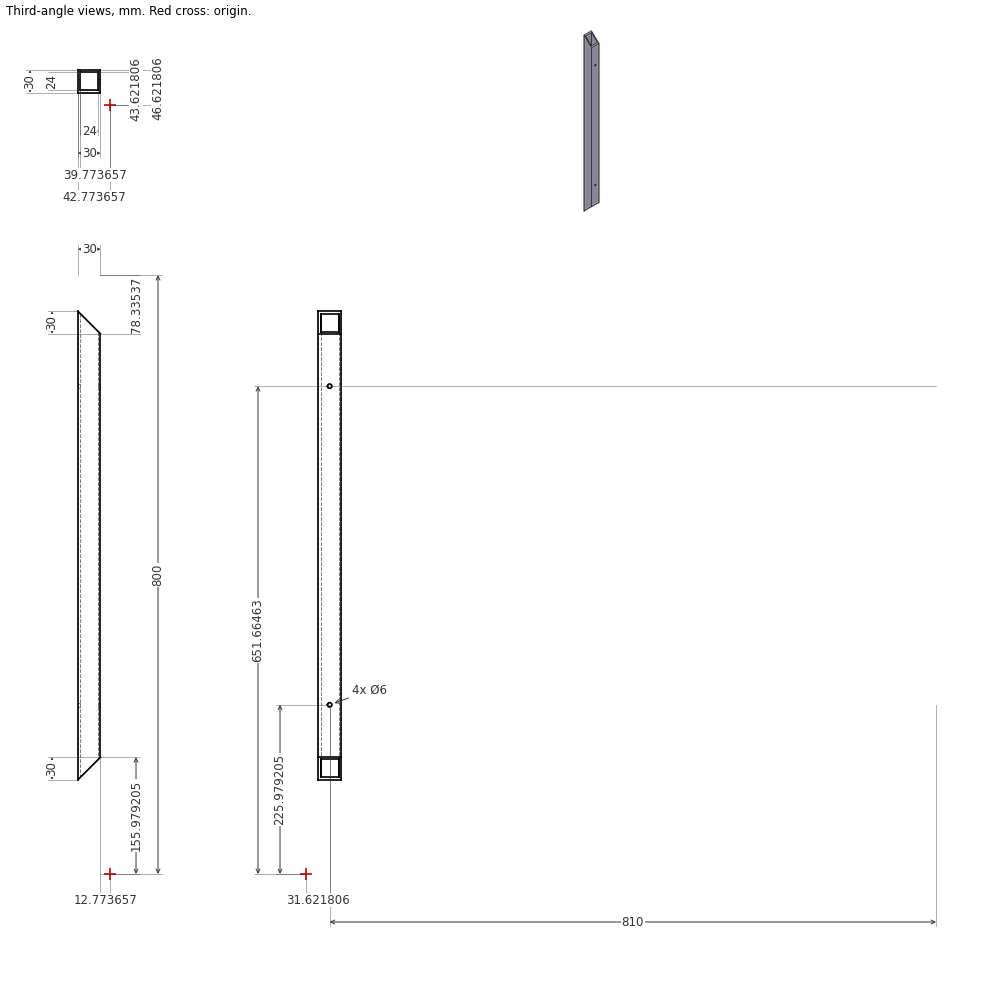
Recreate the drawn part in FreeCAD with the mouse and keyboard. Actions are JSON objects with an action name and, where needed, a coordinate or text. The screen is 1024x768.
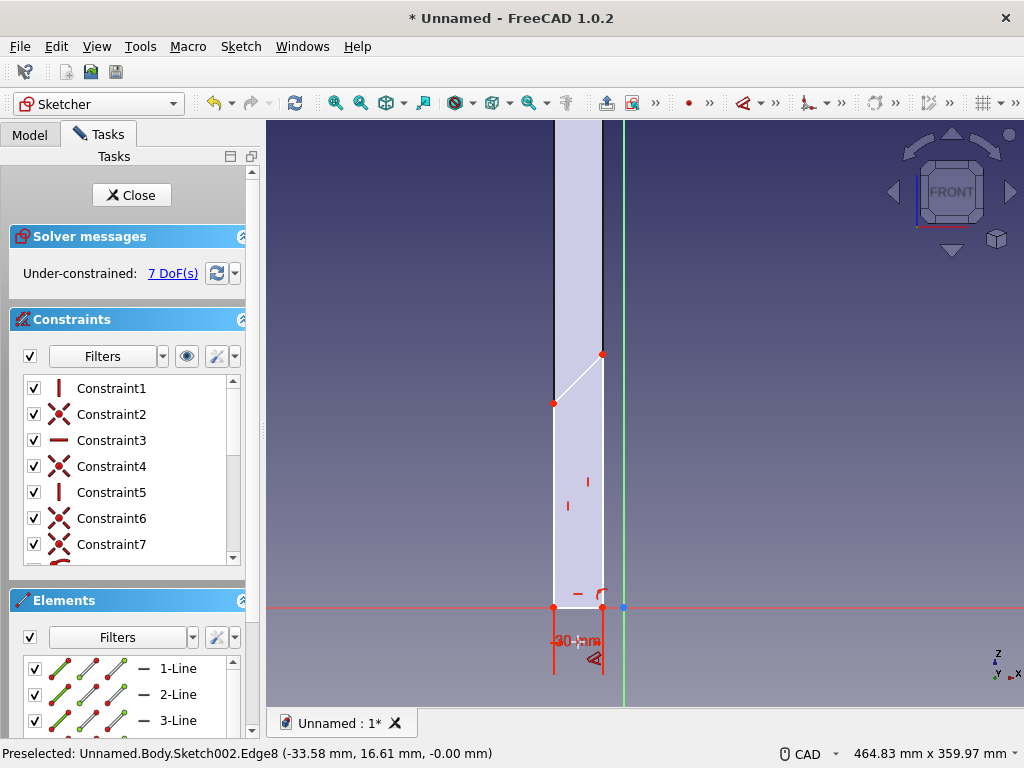
{"action": "scroll", "coordinate": [571, 611], "scroll_direction": "down", "scroll_amount": 6}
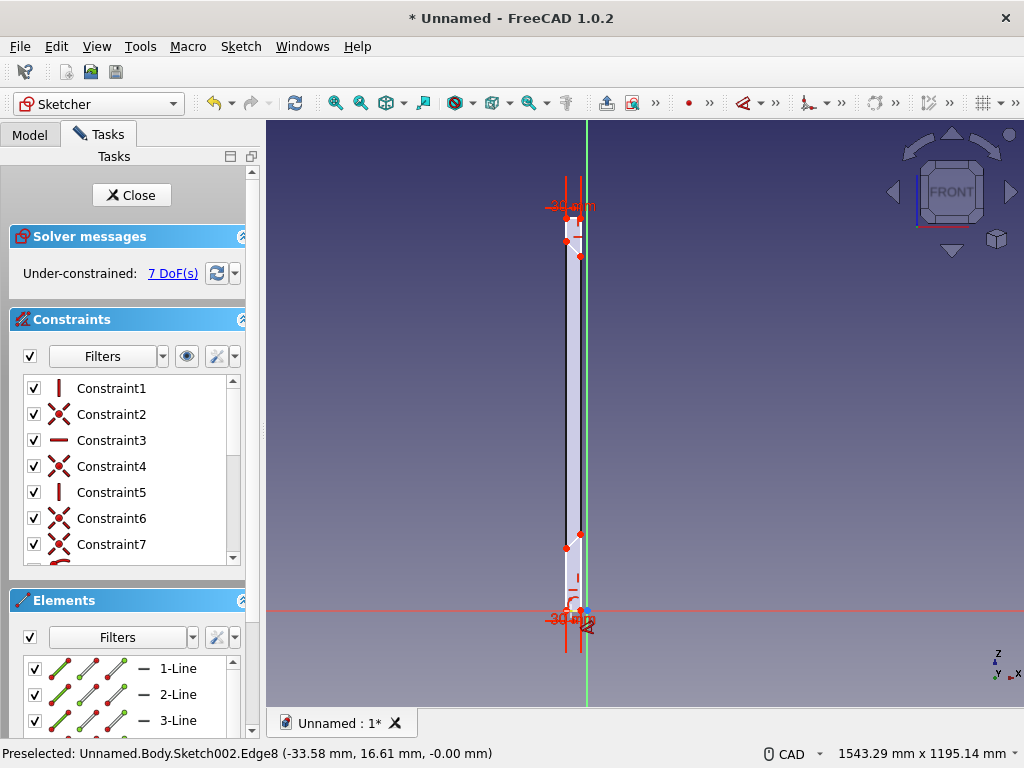
{"action": "scroll", "coordinate": [571, 246], "scroll_direction": "up", "scroll_amount": 5}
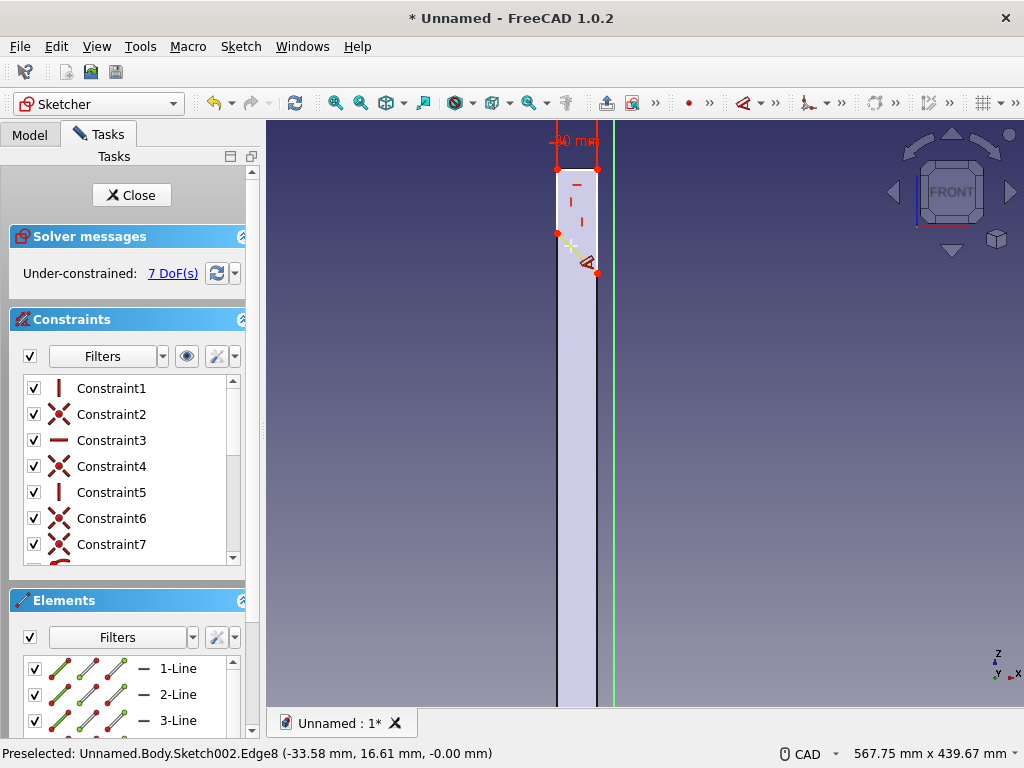
{"action": "left_click", "coordinate": [569, 246]}
{"action": "left_click", "coordinate": [523, 254]}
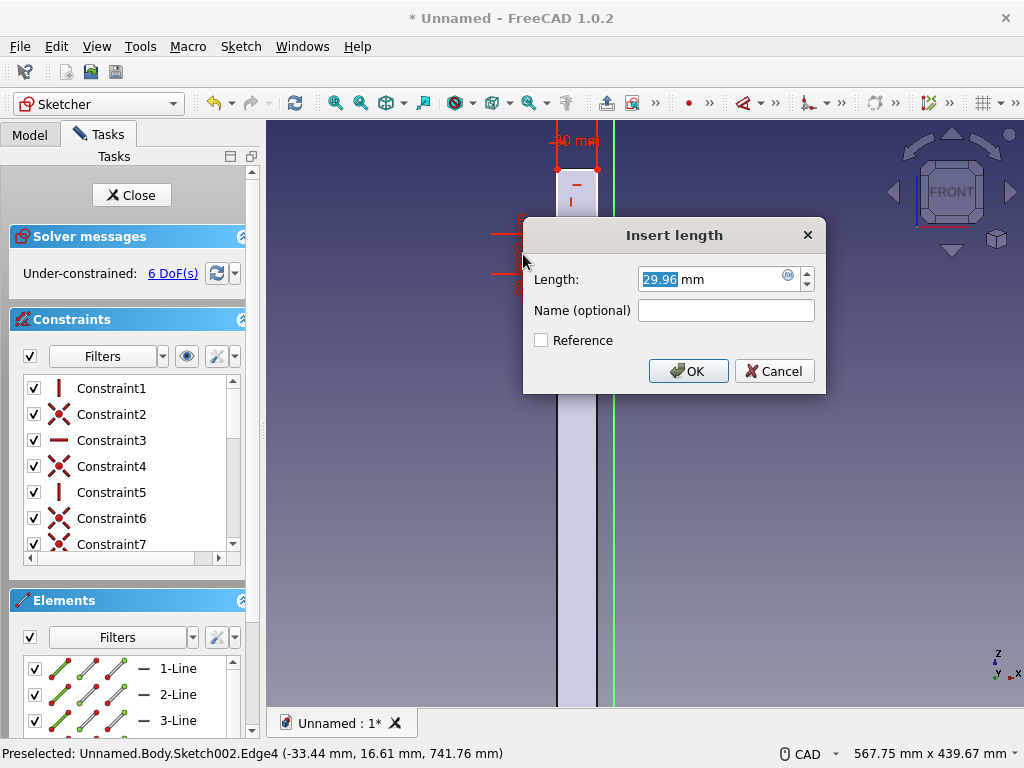
{"action": "type", "text": "30"}
{"action": "key", "text": "Return"}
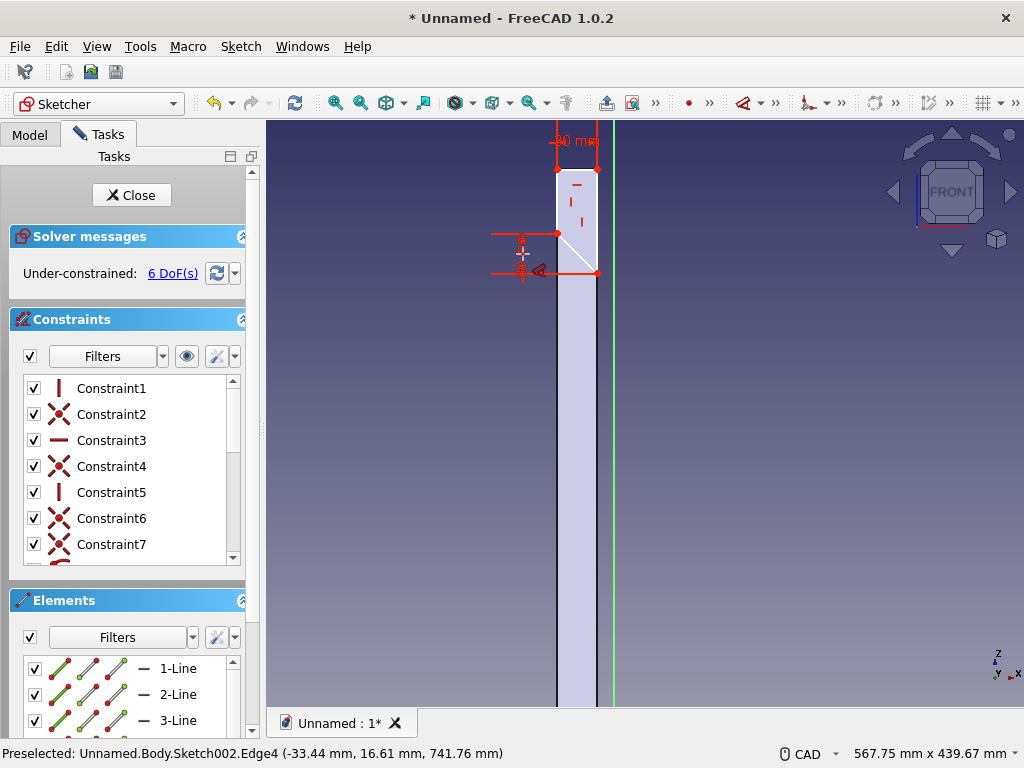
{"action": "scroll", "coordinate": [571, 245], "scroll_direction": "down", "scroll_amount": 5}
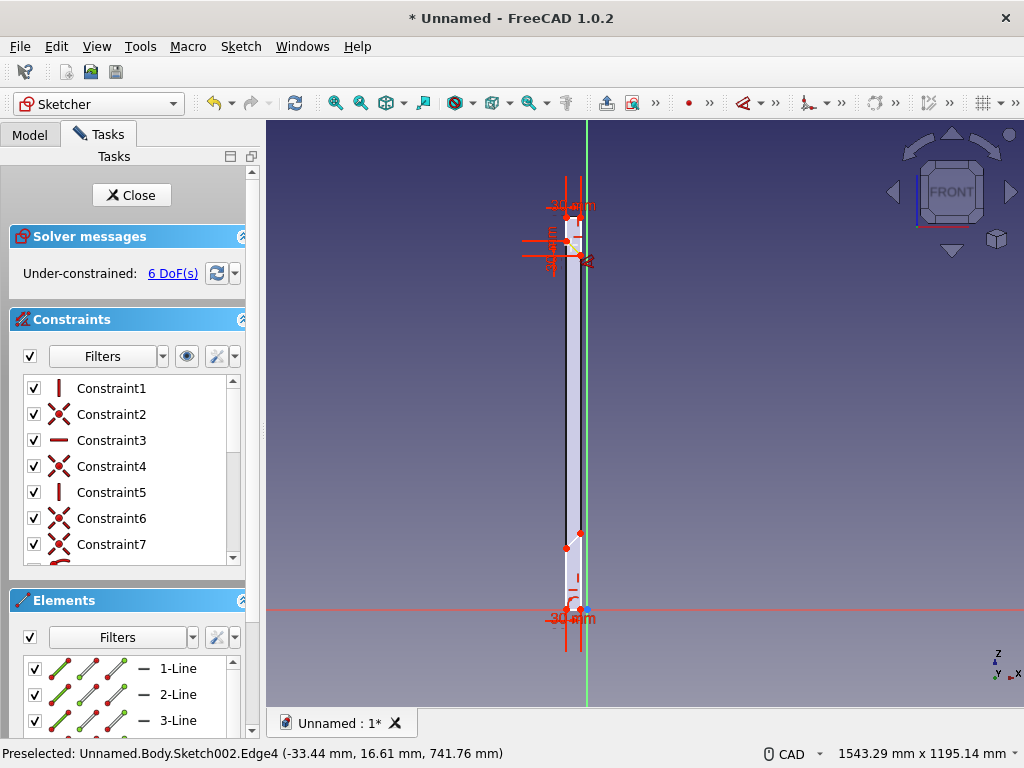
{"action": "scroll", "coordinate": [576, 538], "scroll_direction": "up", "scroll_amount": 6}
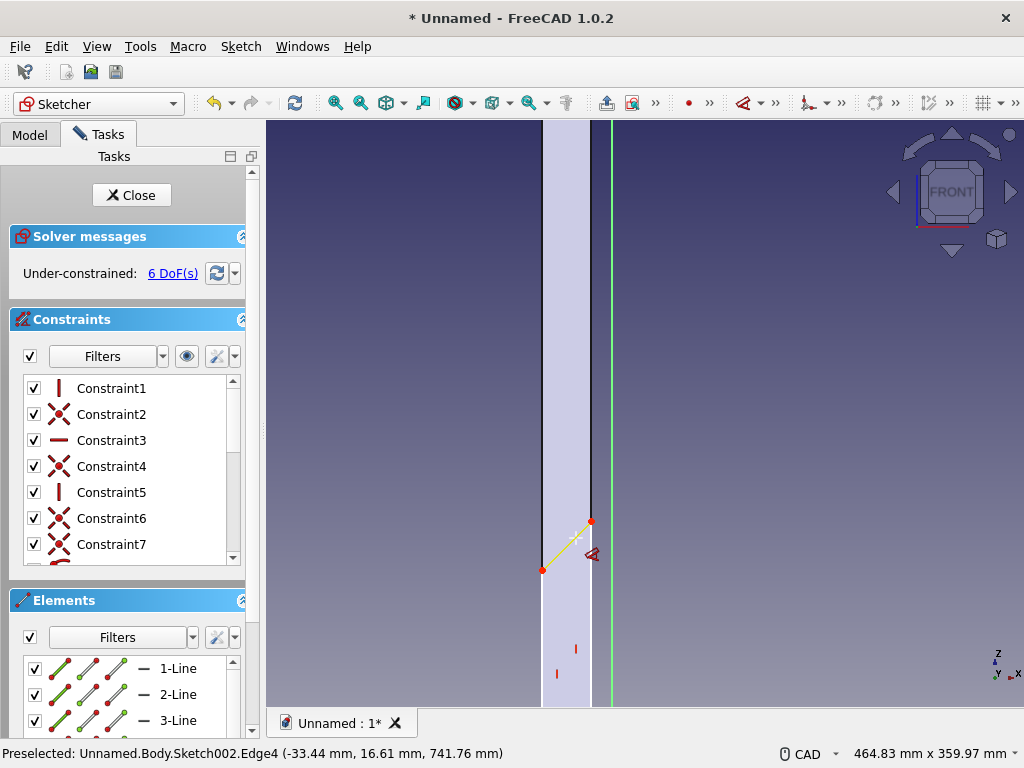
{"action": "left_click", "coordinate": [577, 537]}
{"action": "left_click", "coordinate": [508, 546]}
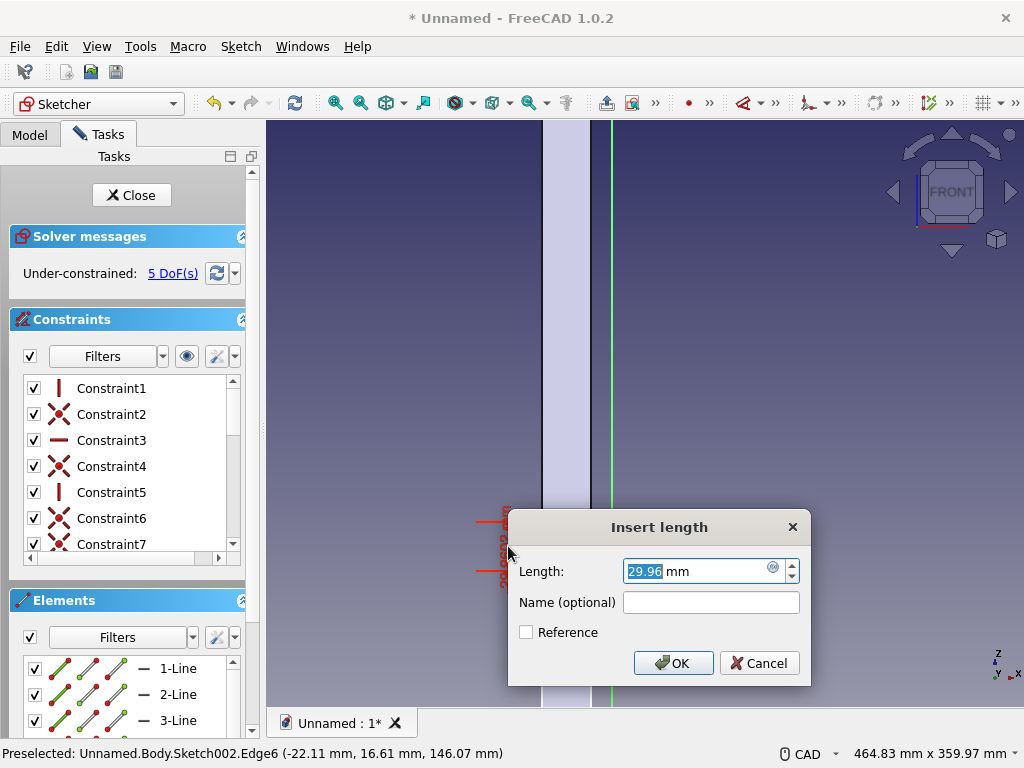
{"action": "type", "text": "30"}
{"action": "key", "text": "Return"}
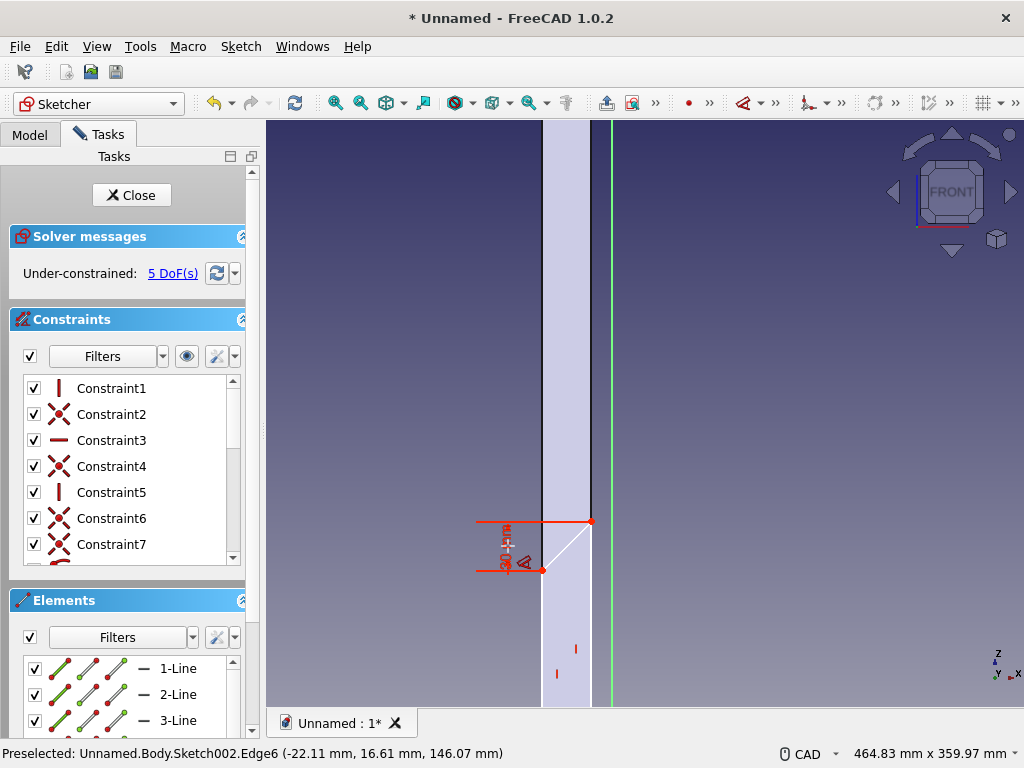
{"action": "scroll", "coordinate": [576, 539], "scroll_direction": "down", "scroll_amount": 6}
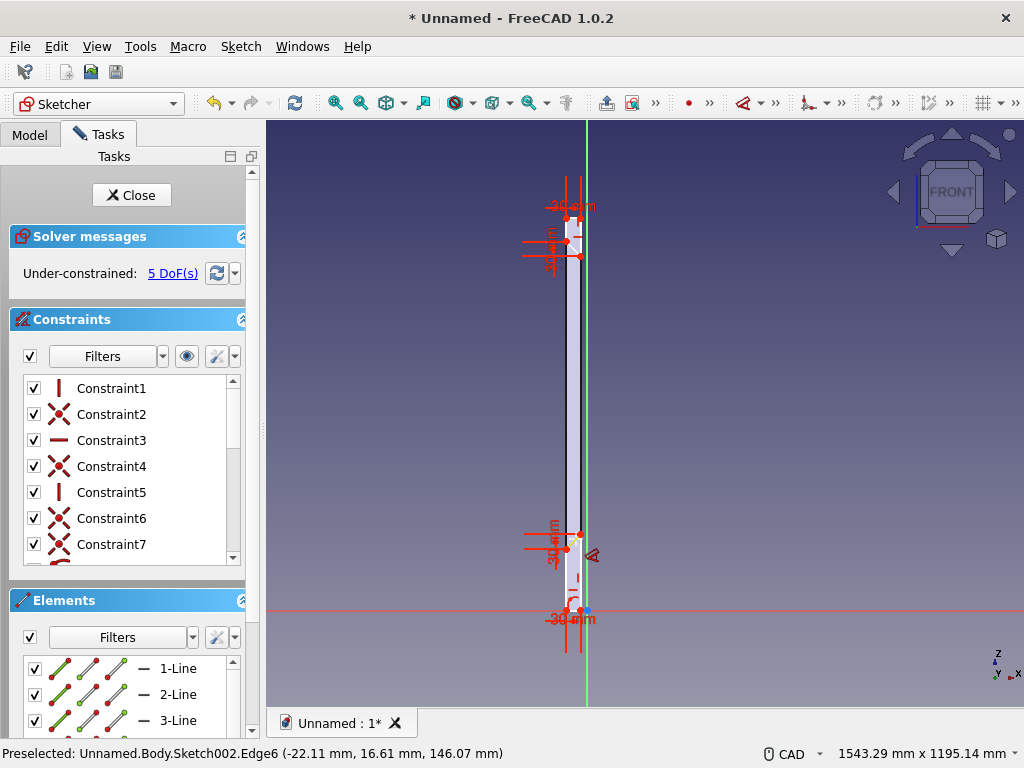
{"action": "left_click", "coordinate": [581, 218]}
{"action": "left_click", "coordinate": [621, 414]}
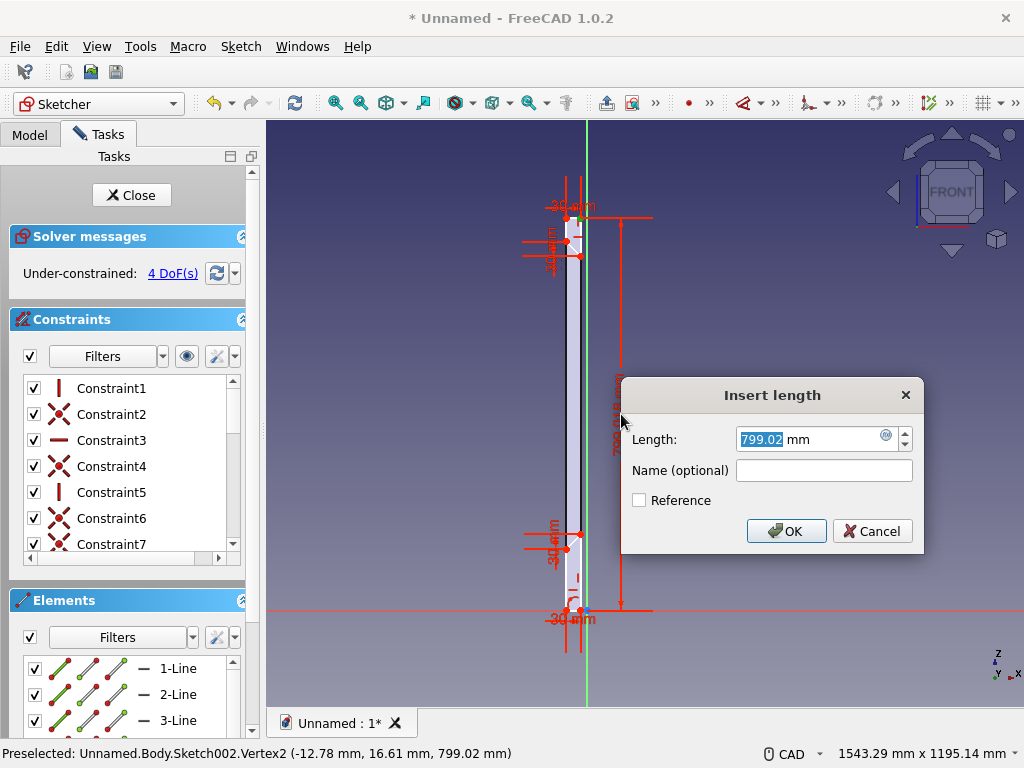
{"action": "type", "text": "800"}
{"action": "key", "text": "Return"}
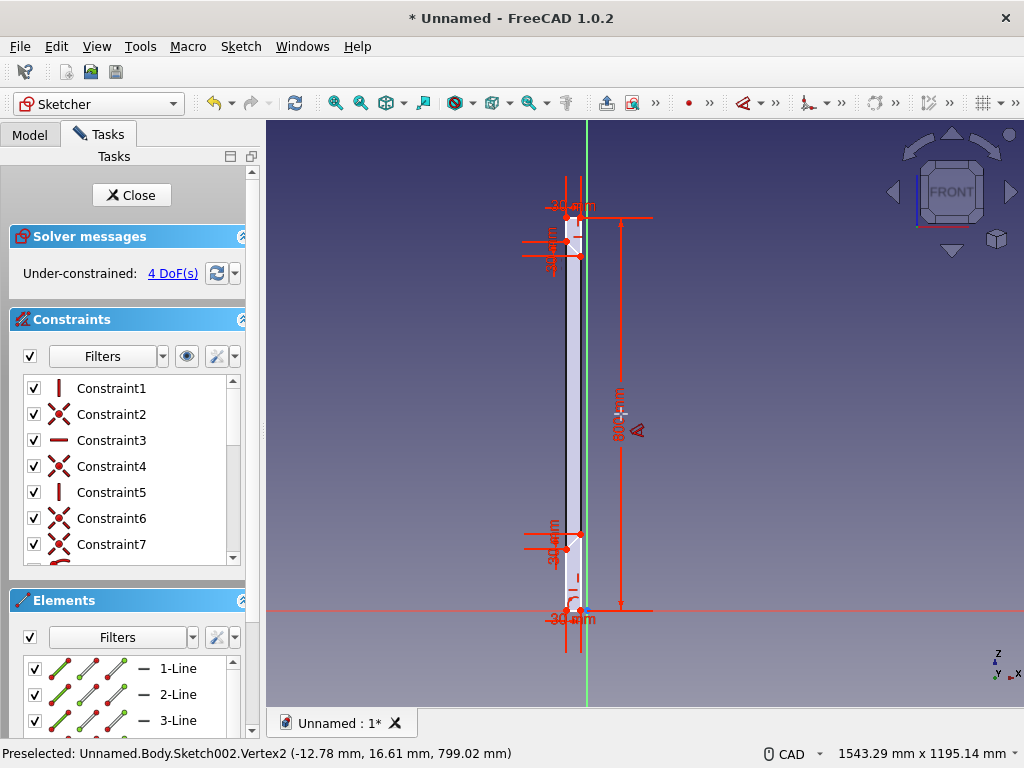
{"action": "scroll", "coordinate": [581, 245], "scroll_direction": "up", "scroll_amount": 4}